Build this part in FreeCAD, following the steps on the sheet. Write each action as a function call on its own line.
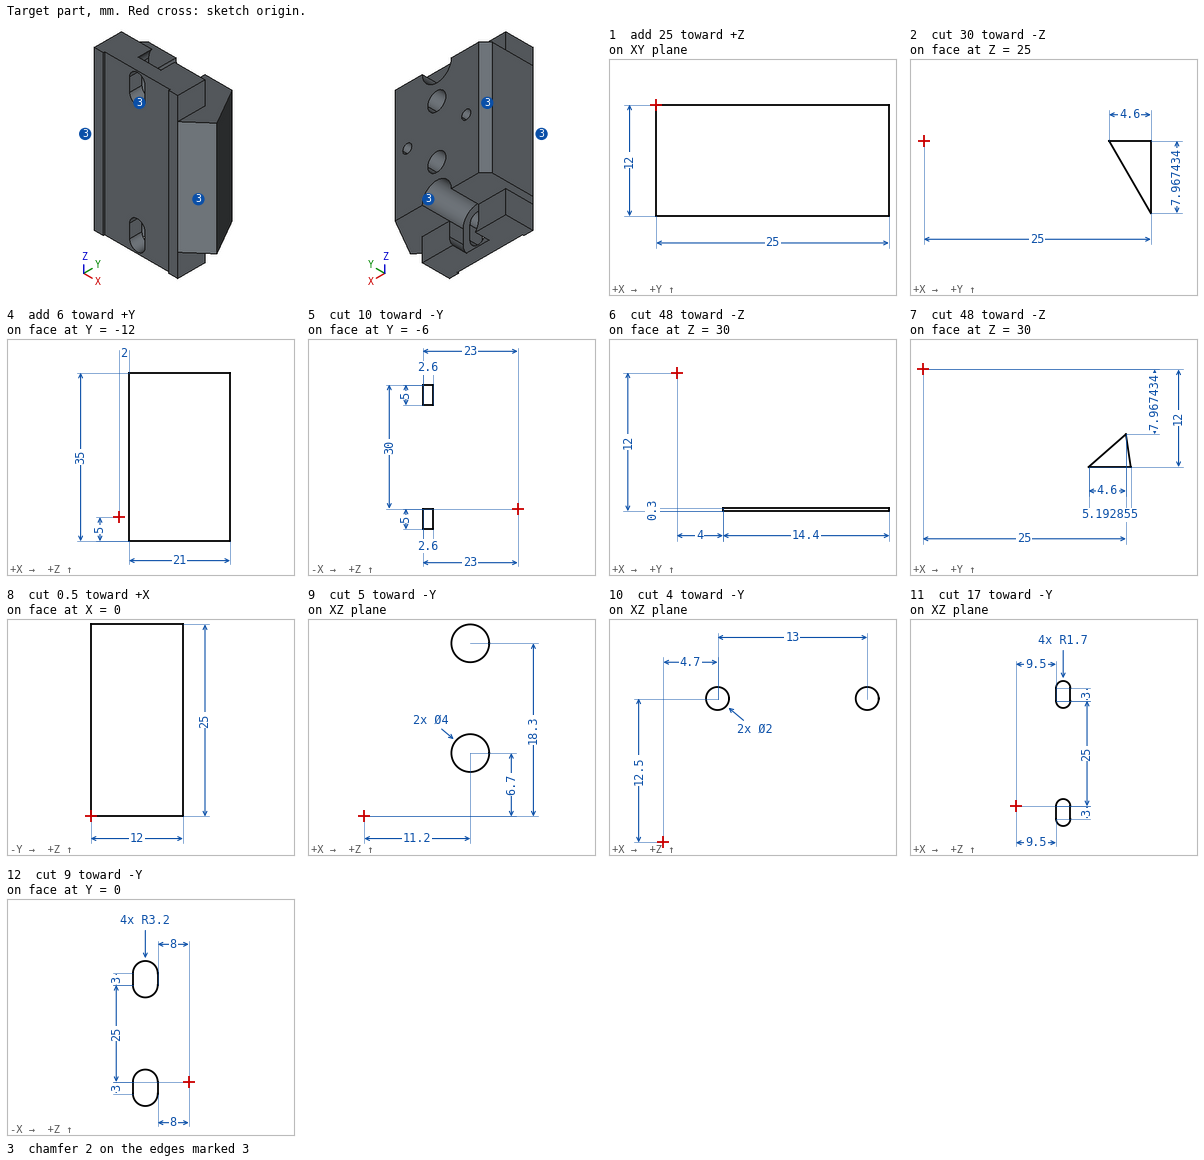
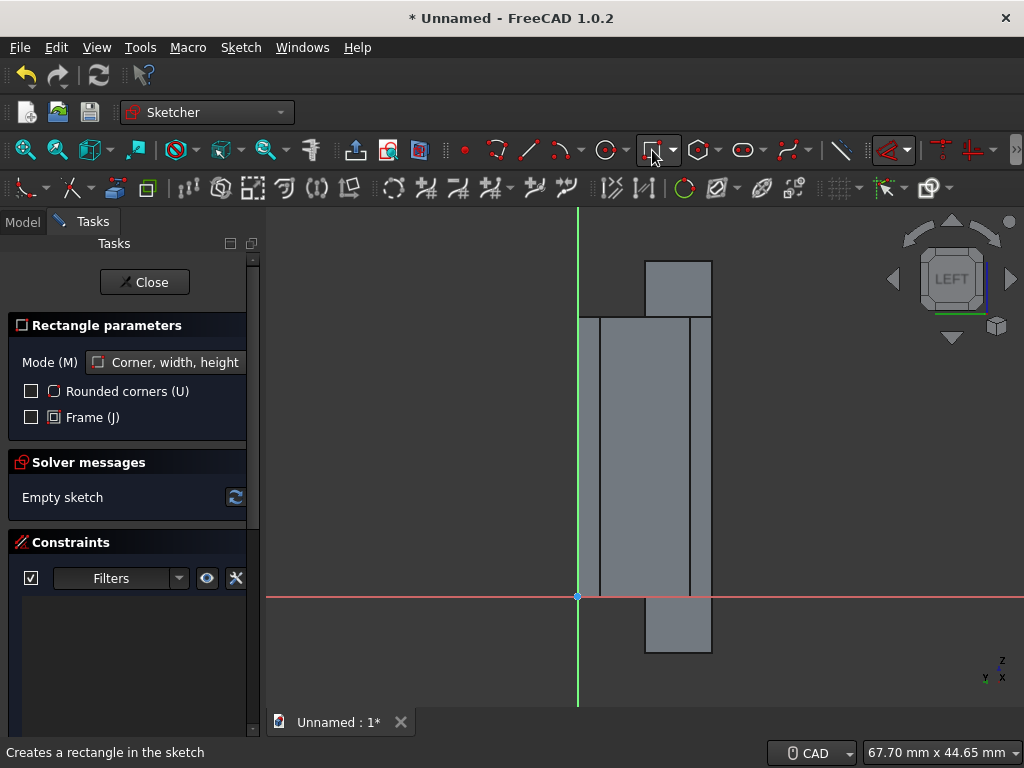
click(578, 597)
click(712, 317)
key(Escape)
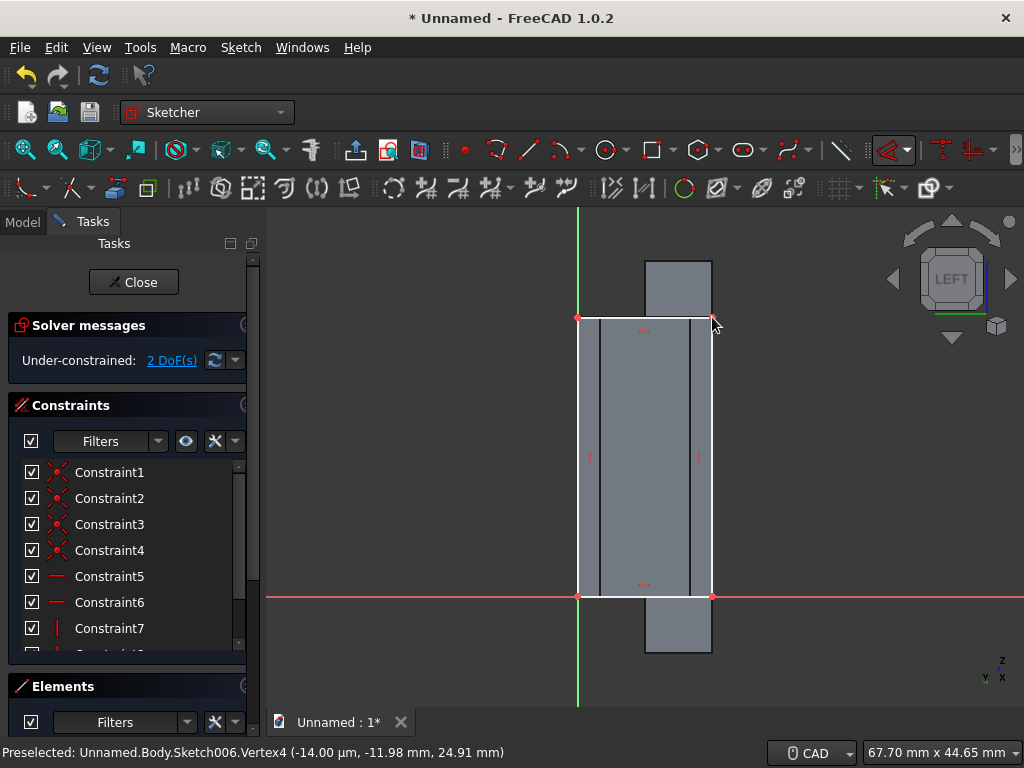
click(618, 597)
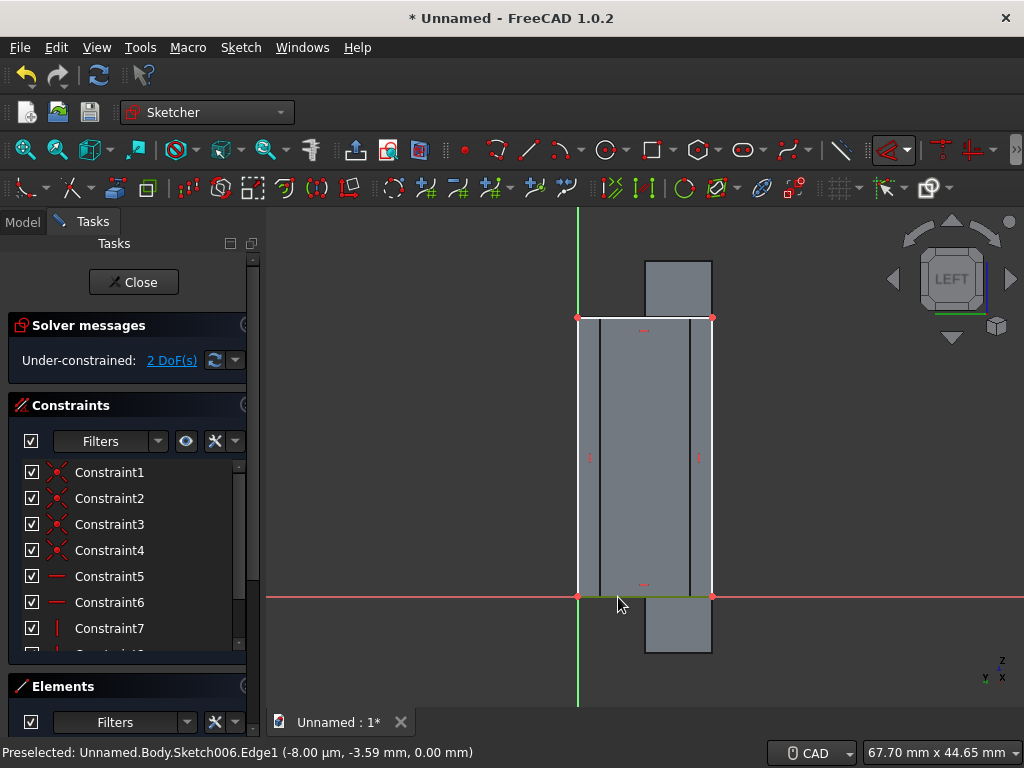
key(l)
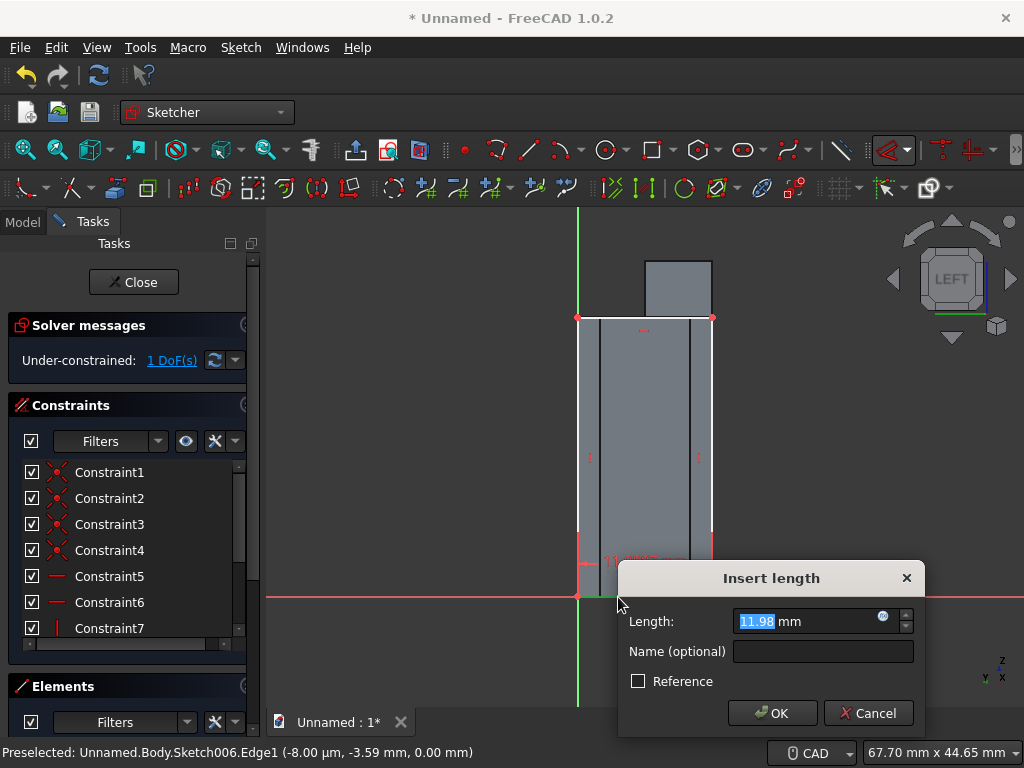
text(12)
key(Return)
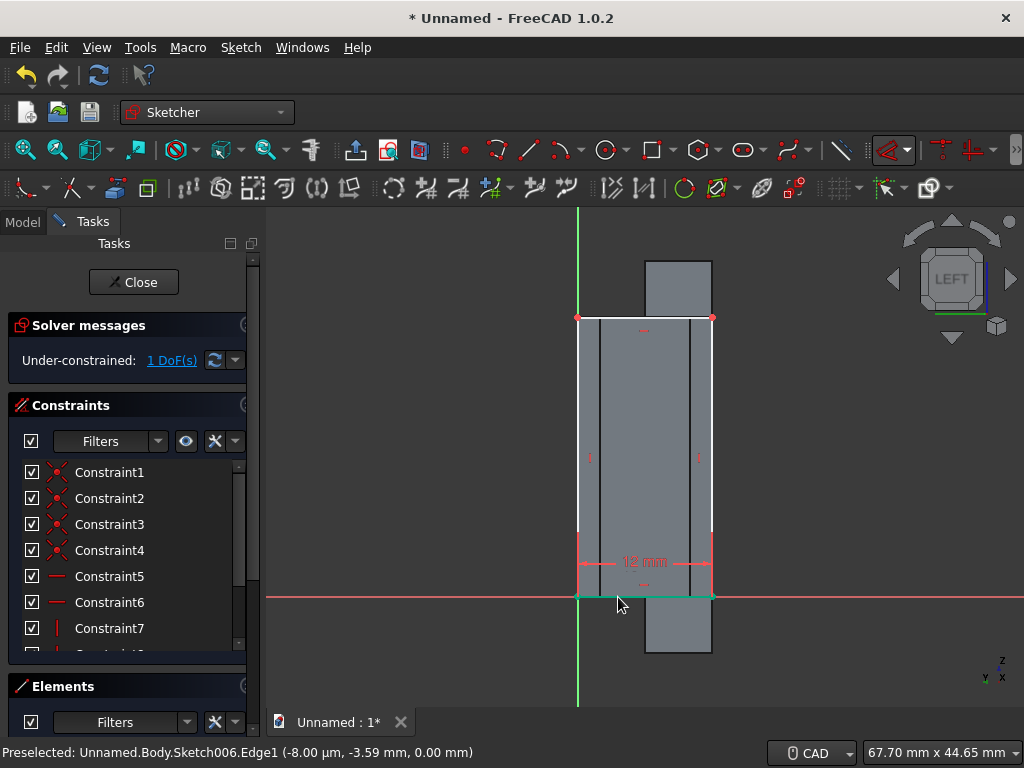
click(712, 513)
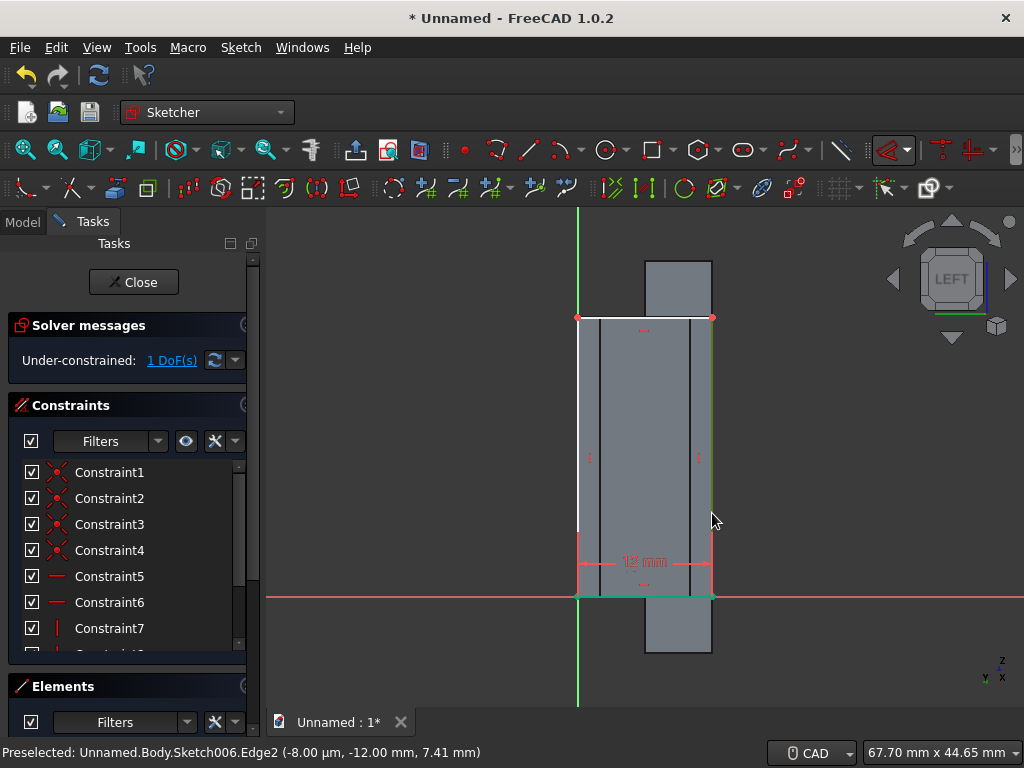
key(i)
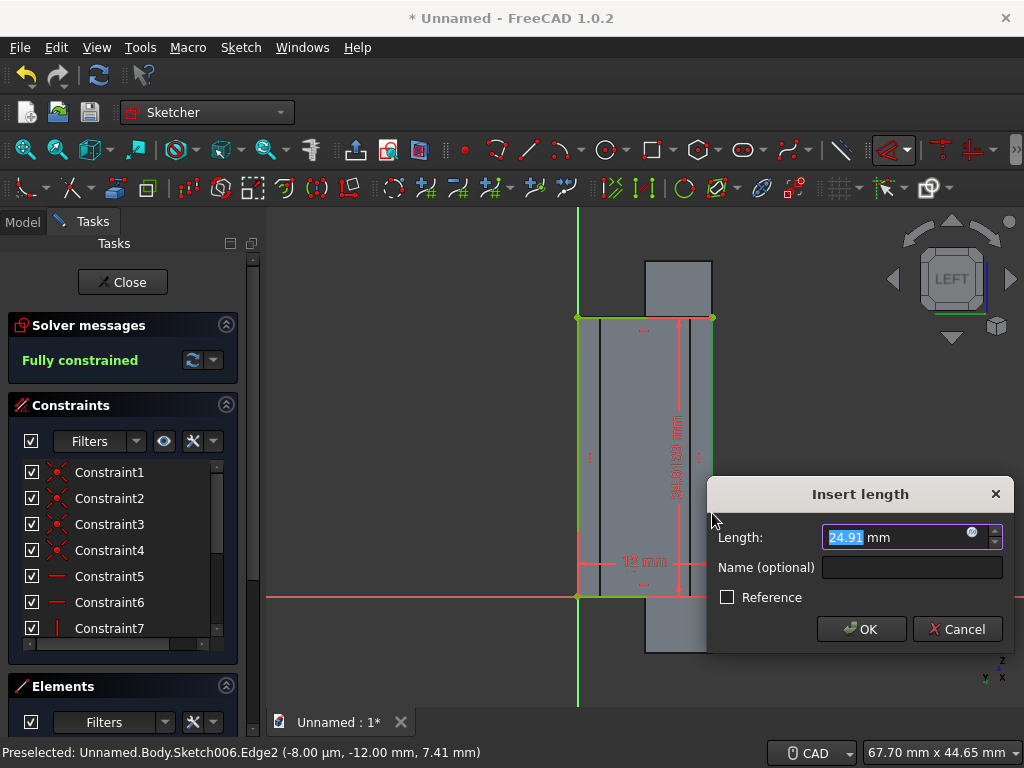
text(25)
key(Return)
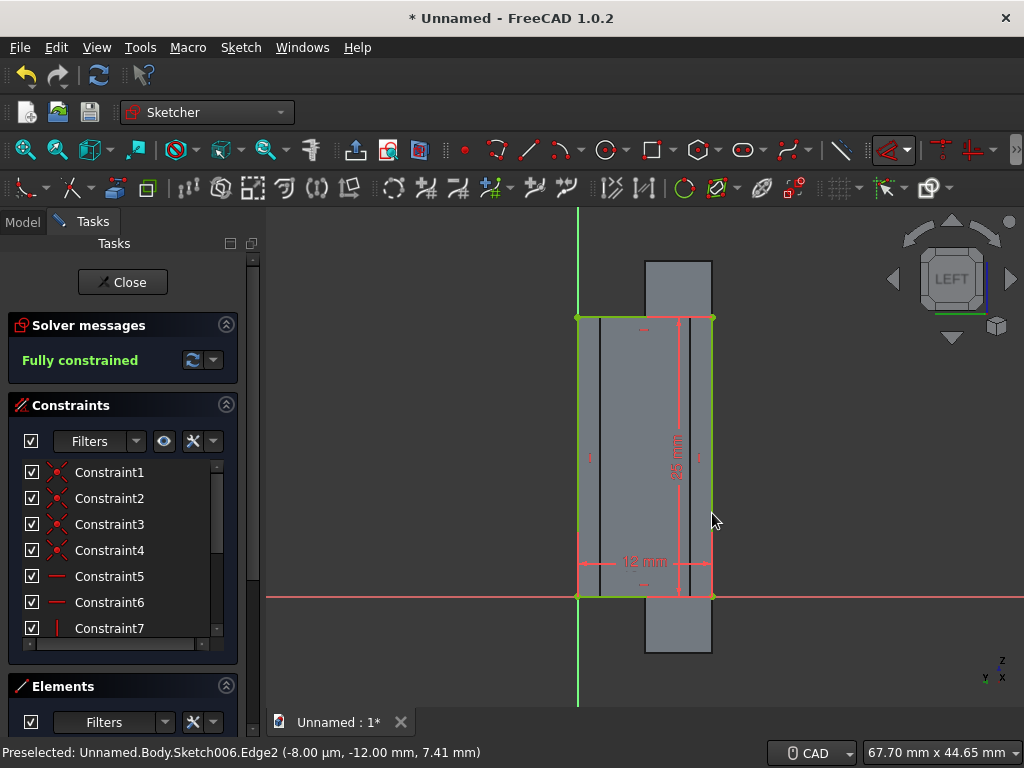
click(123, 282)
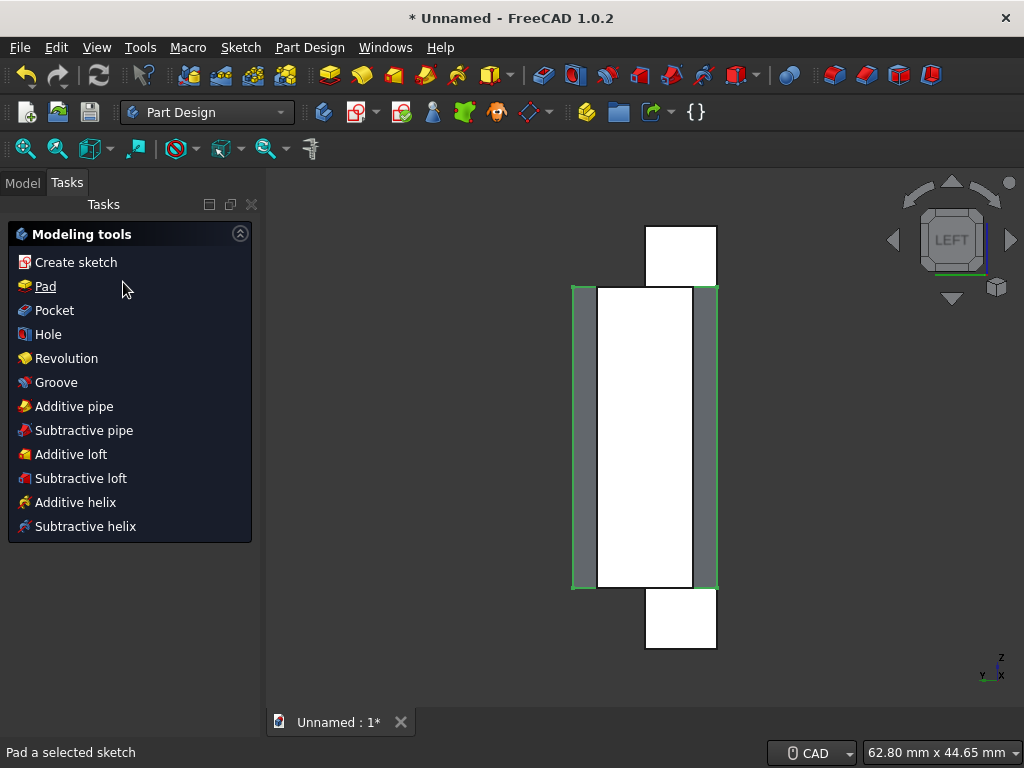
click(544, 76)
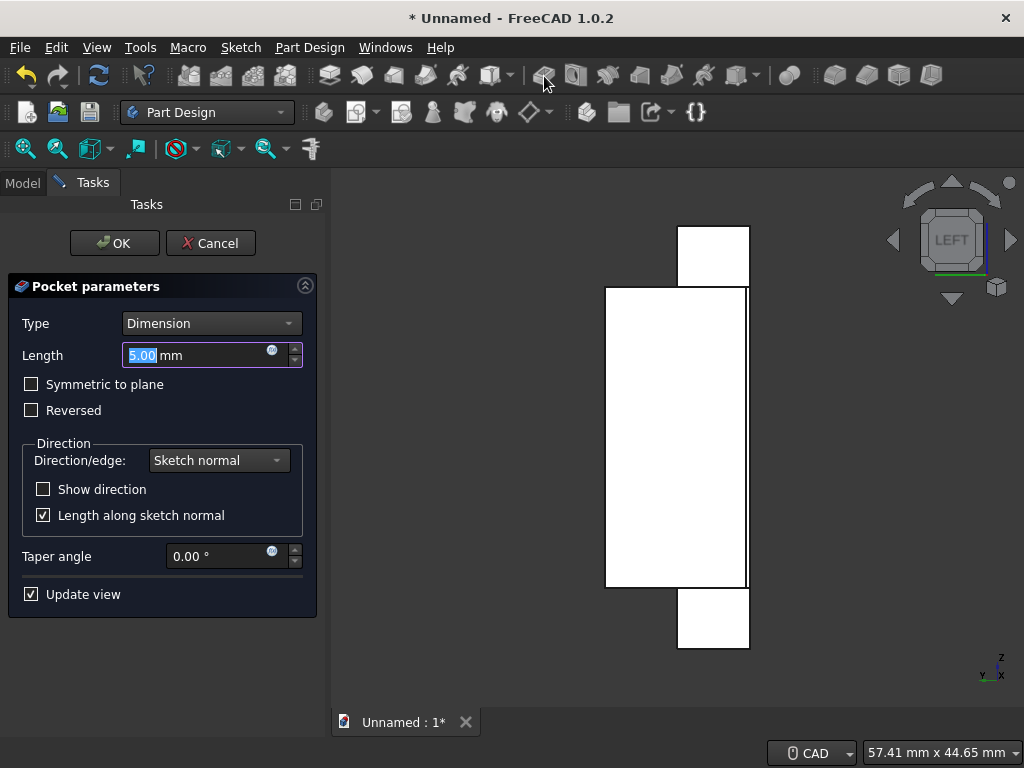
text(0.5)
key(Tab)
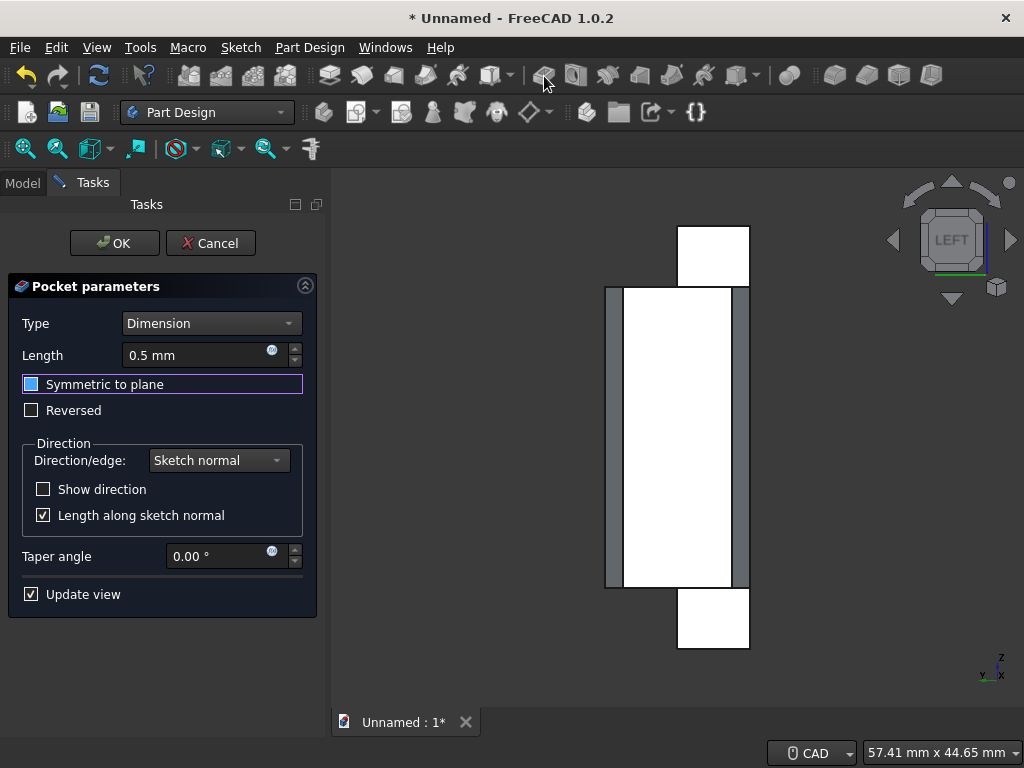
click(115, 243)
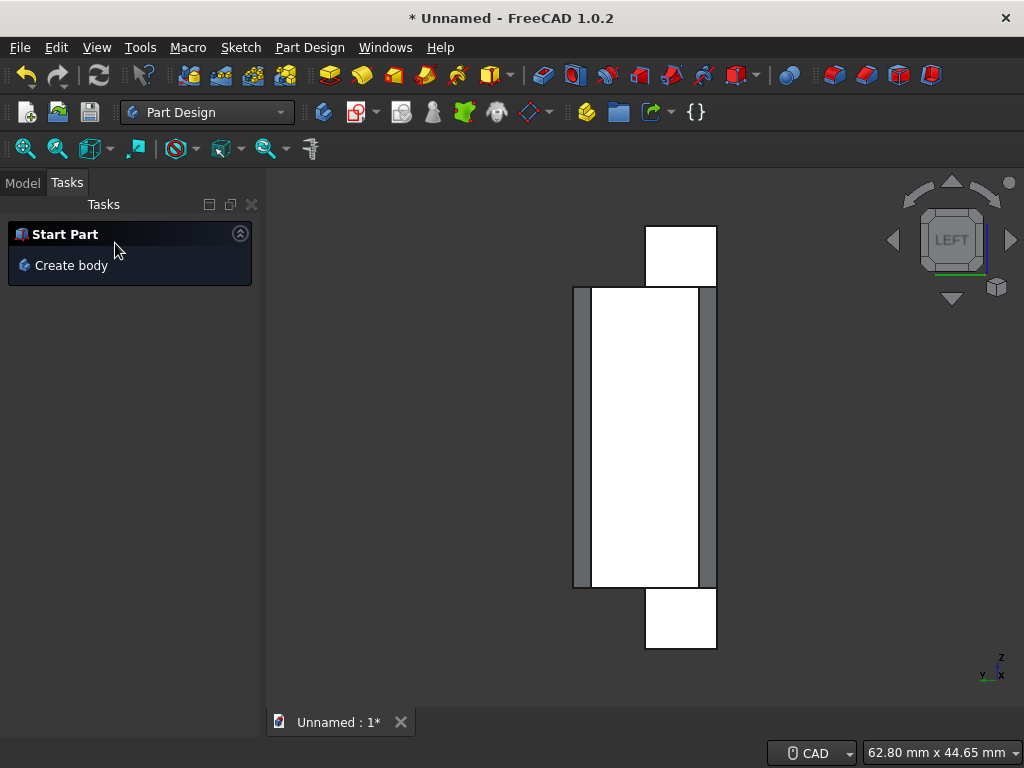
click(356, 112)